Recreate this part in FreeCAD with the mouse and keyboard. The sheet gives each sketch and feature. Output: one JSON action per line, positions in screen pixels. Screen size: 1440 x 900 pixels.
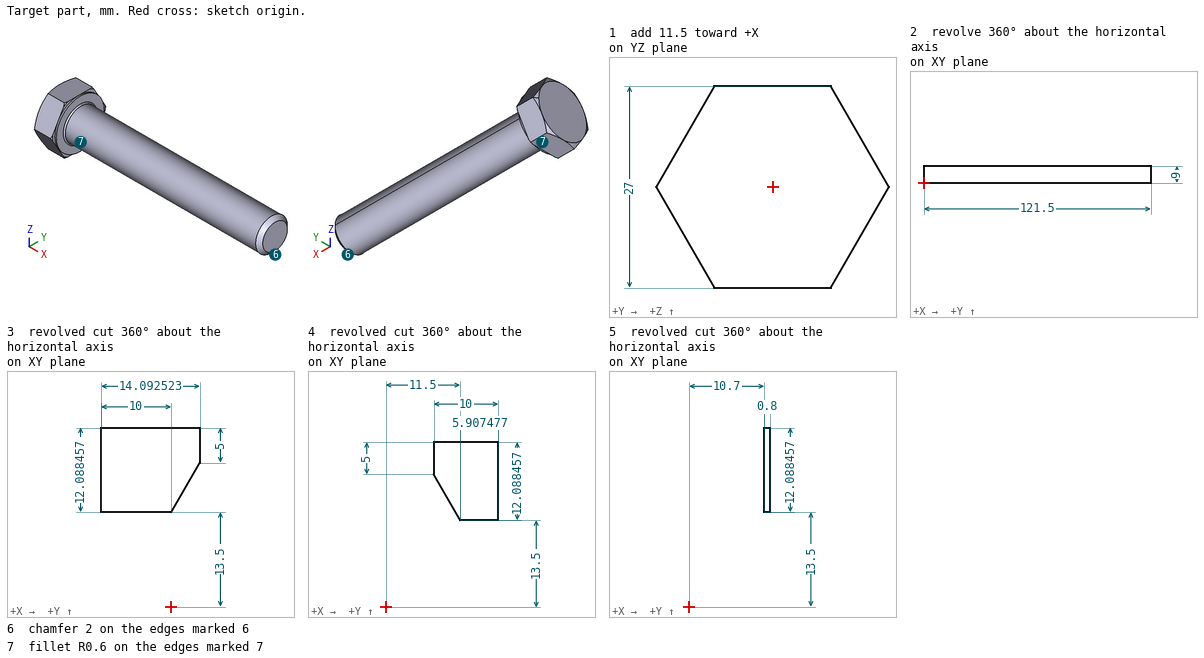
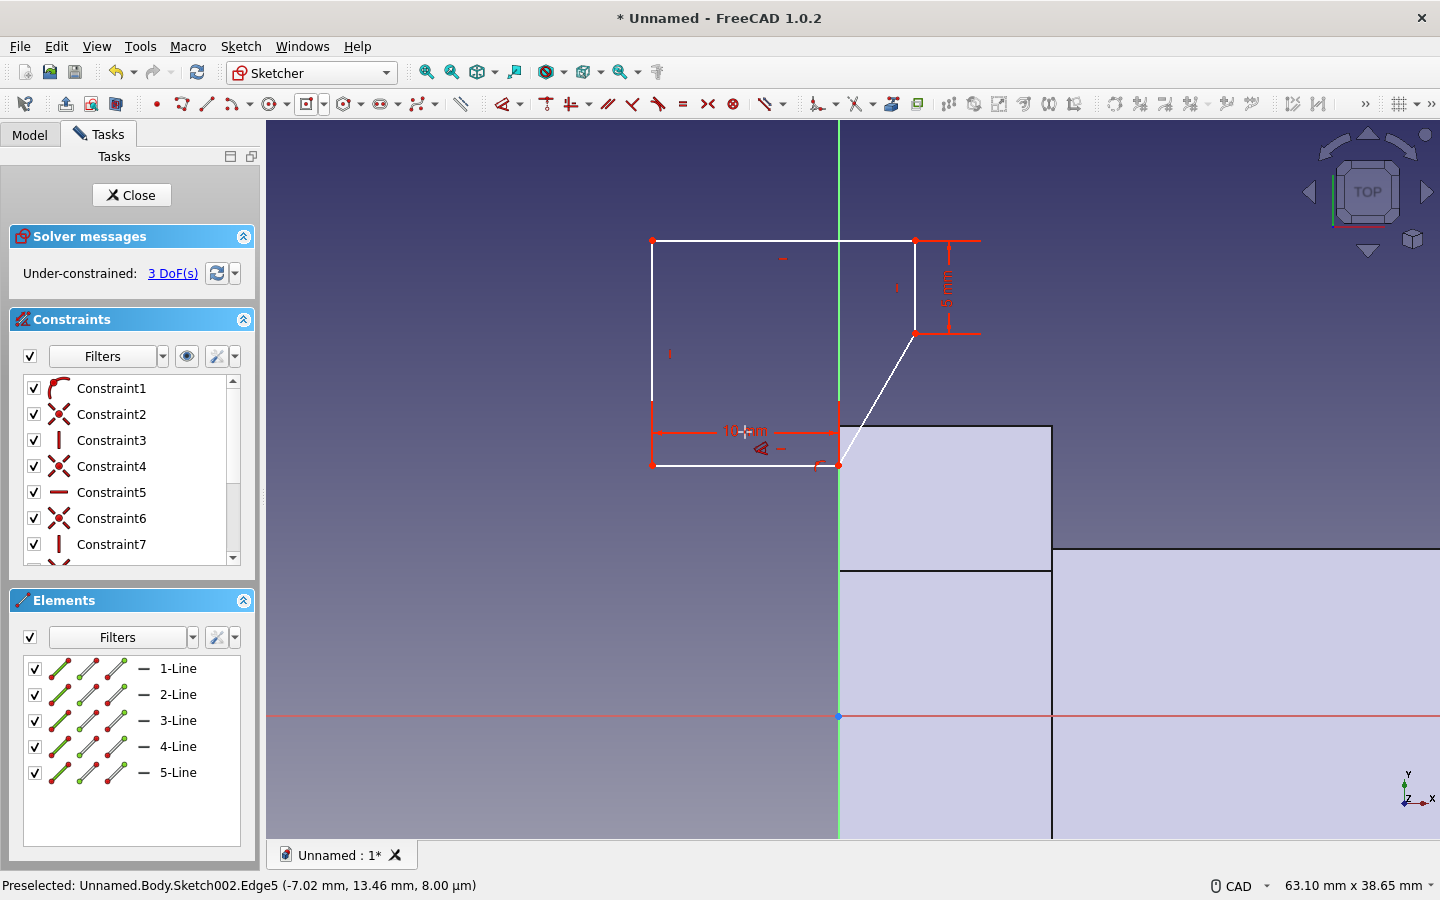
{"action": "left_click", "coordinate": [839, 466]}
{"action": "left_click", "coordinate": [873, 591]}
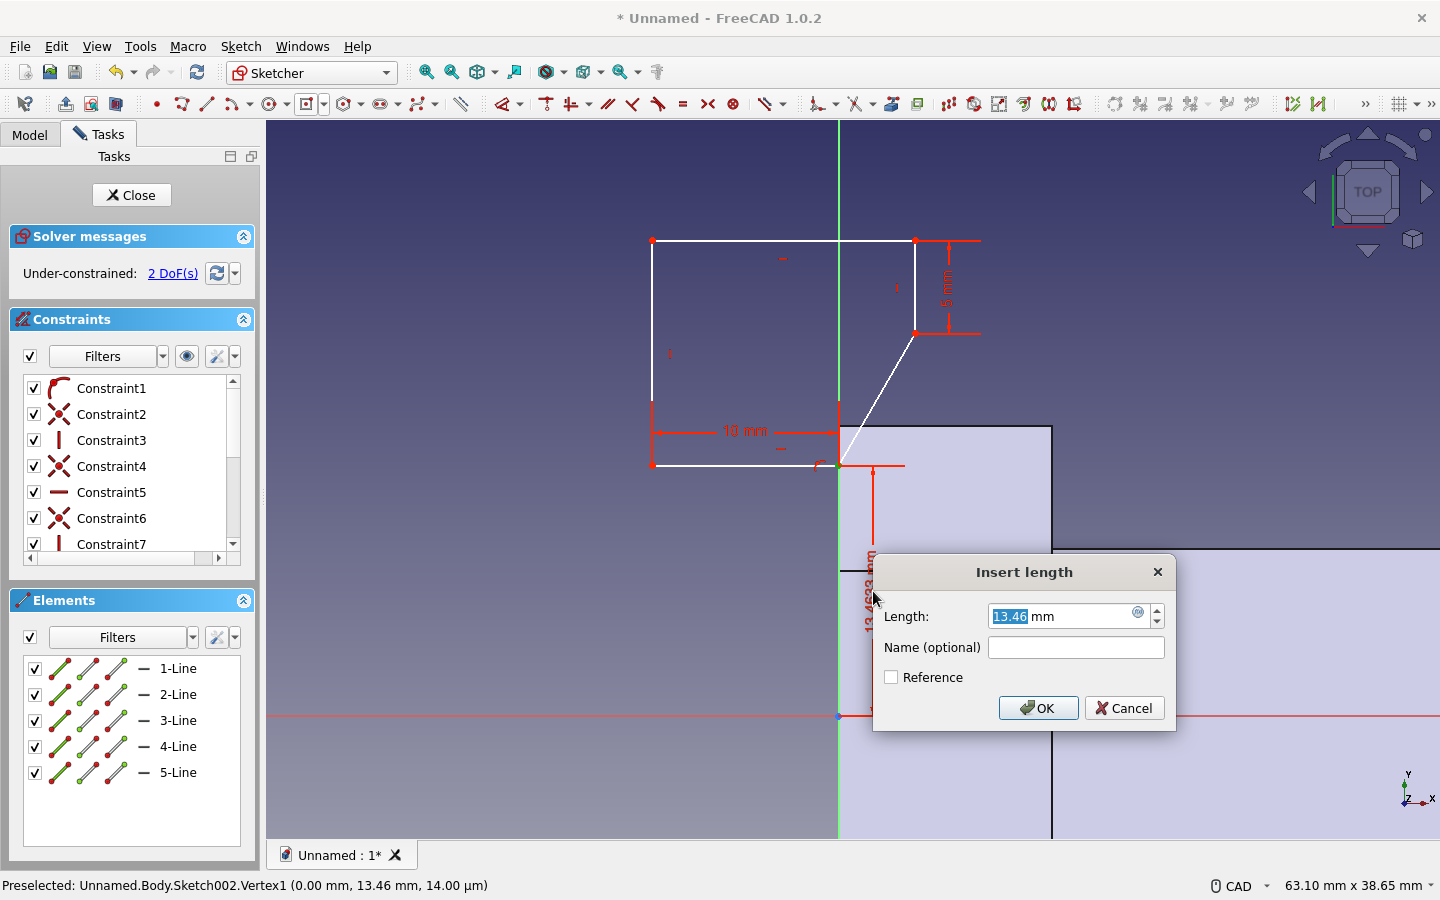
{"action": "type", "text": "13.5"}
{"action": "key", "text": "Return"}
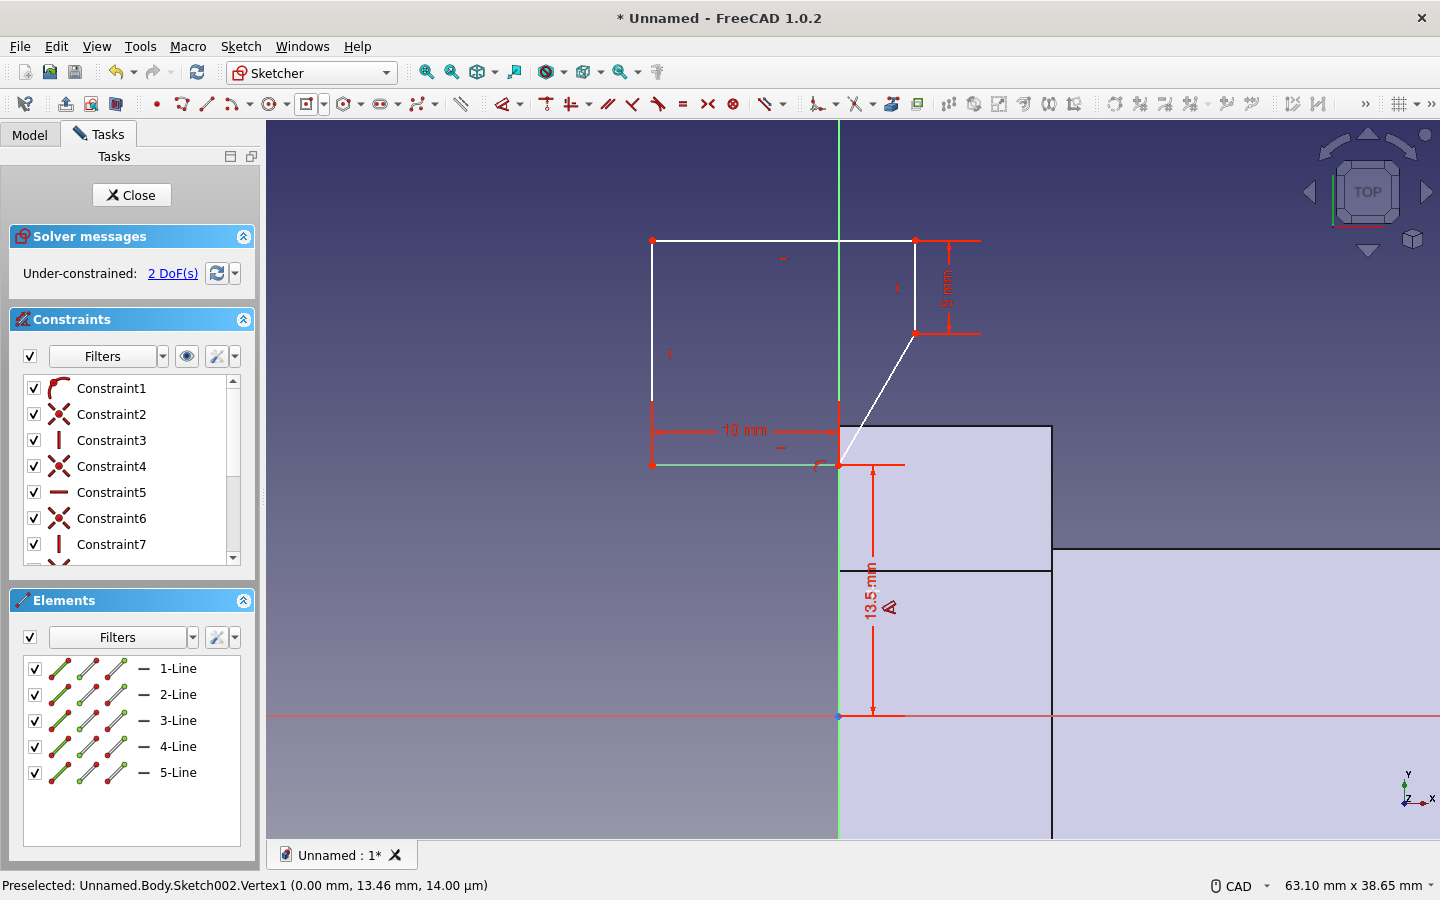
{"action": "left_click", "coordinate": [836, 241]}
{"action": "left_click", "coordinate": [784, 207]}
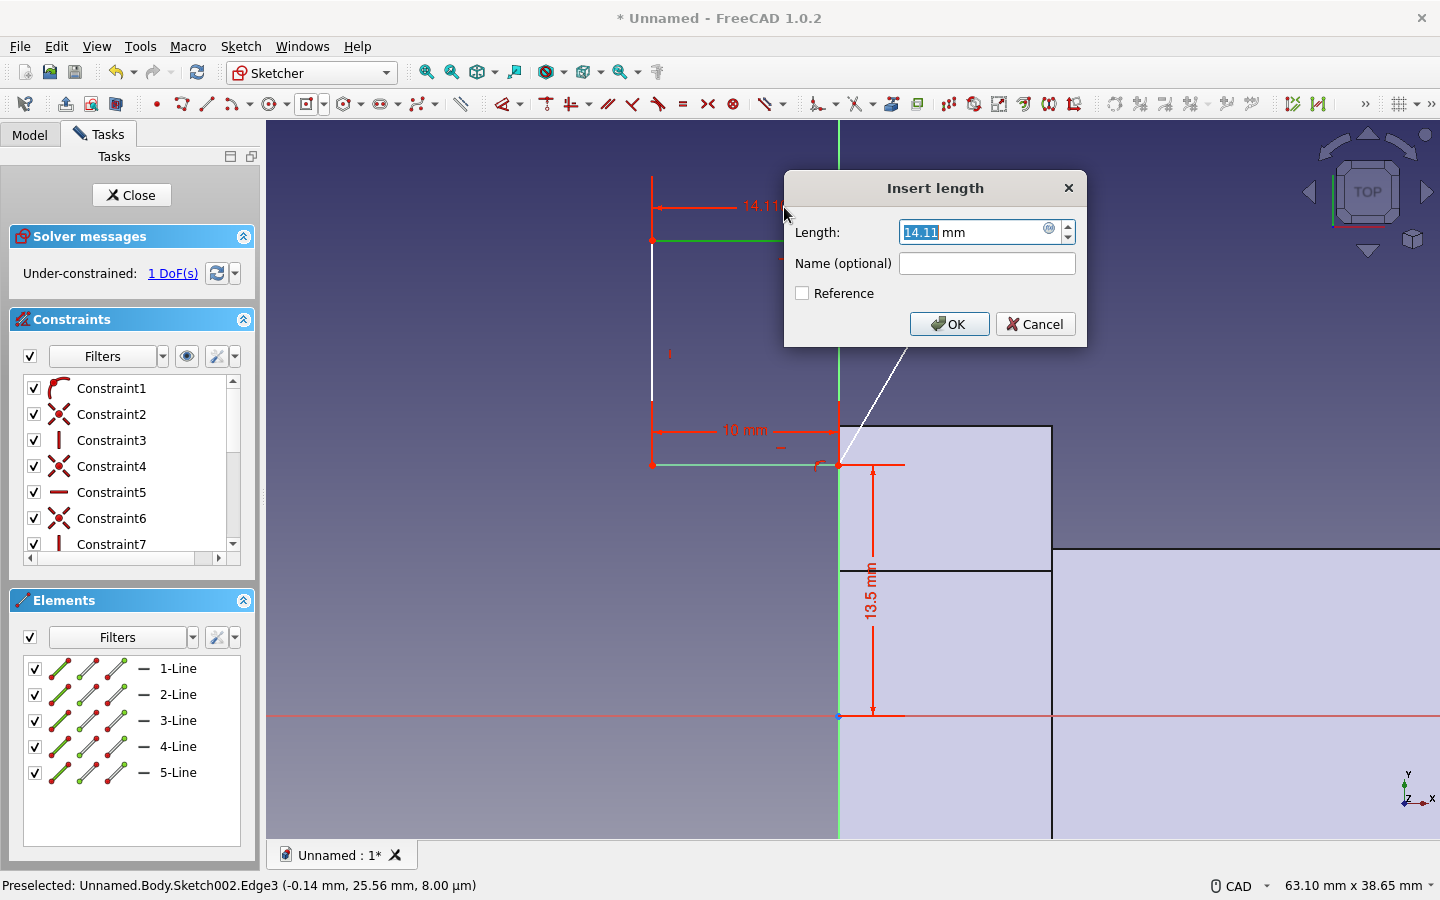
{"action": "type", "text": "14.092523"}
{"action": "key", "text": "Return"}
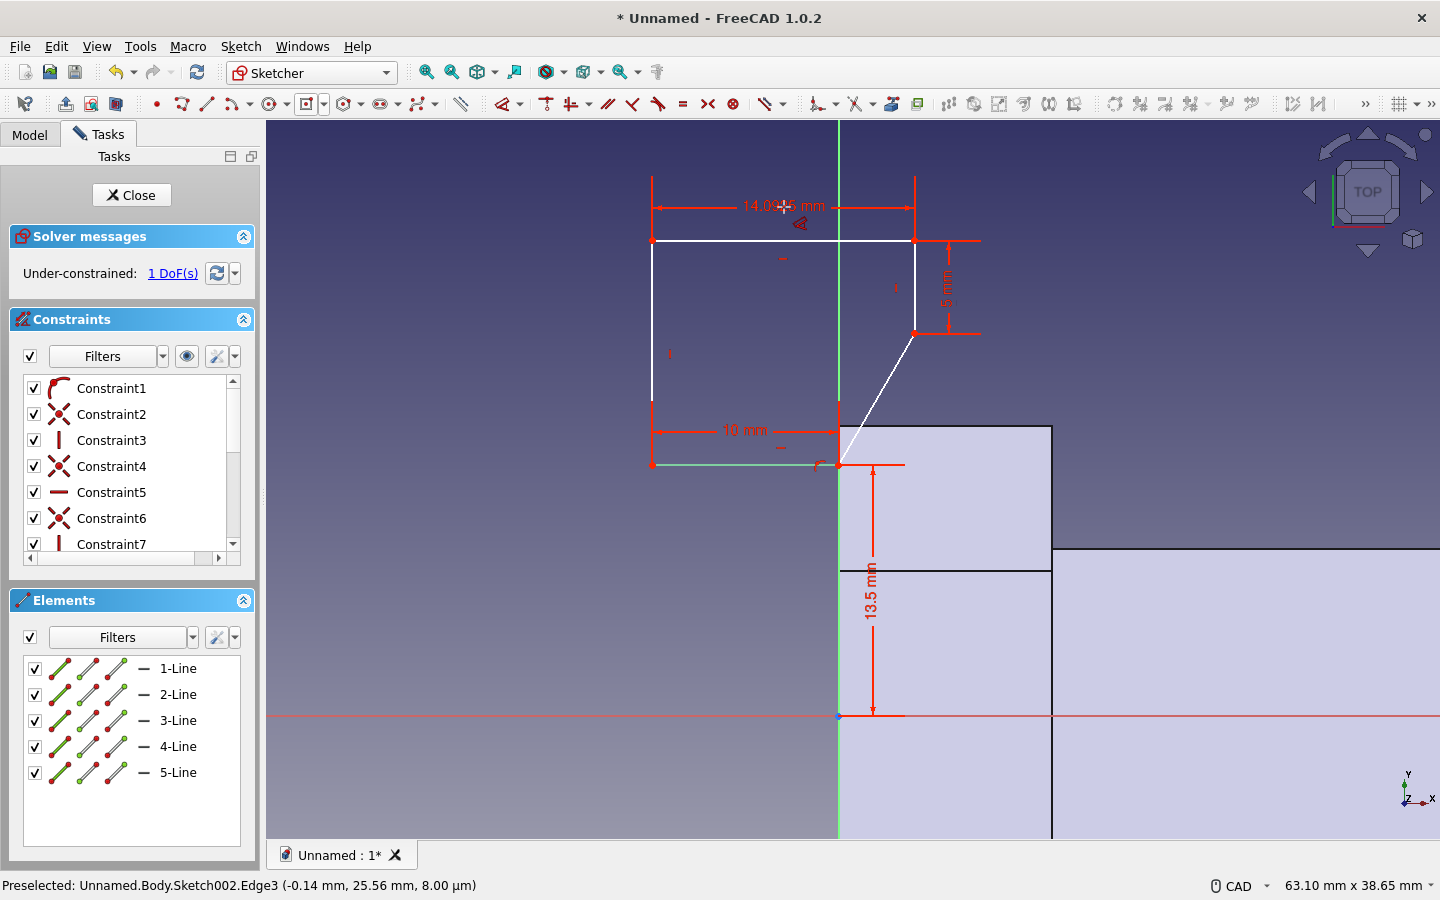
{"action": "left_click", "coordinate": [652, 308]}
{"action": "left_click", "coordinate": [618, 353]}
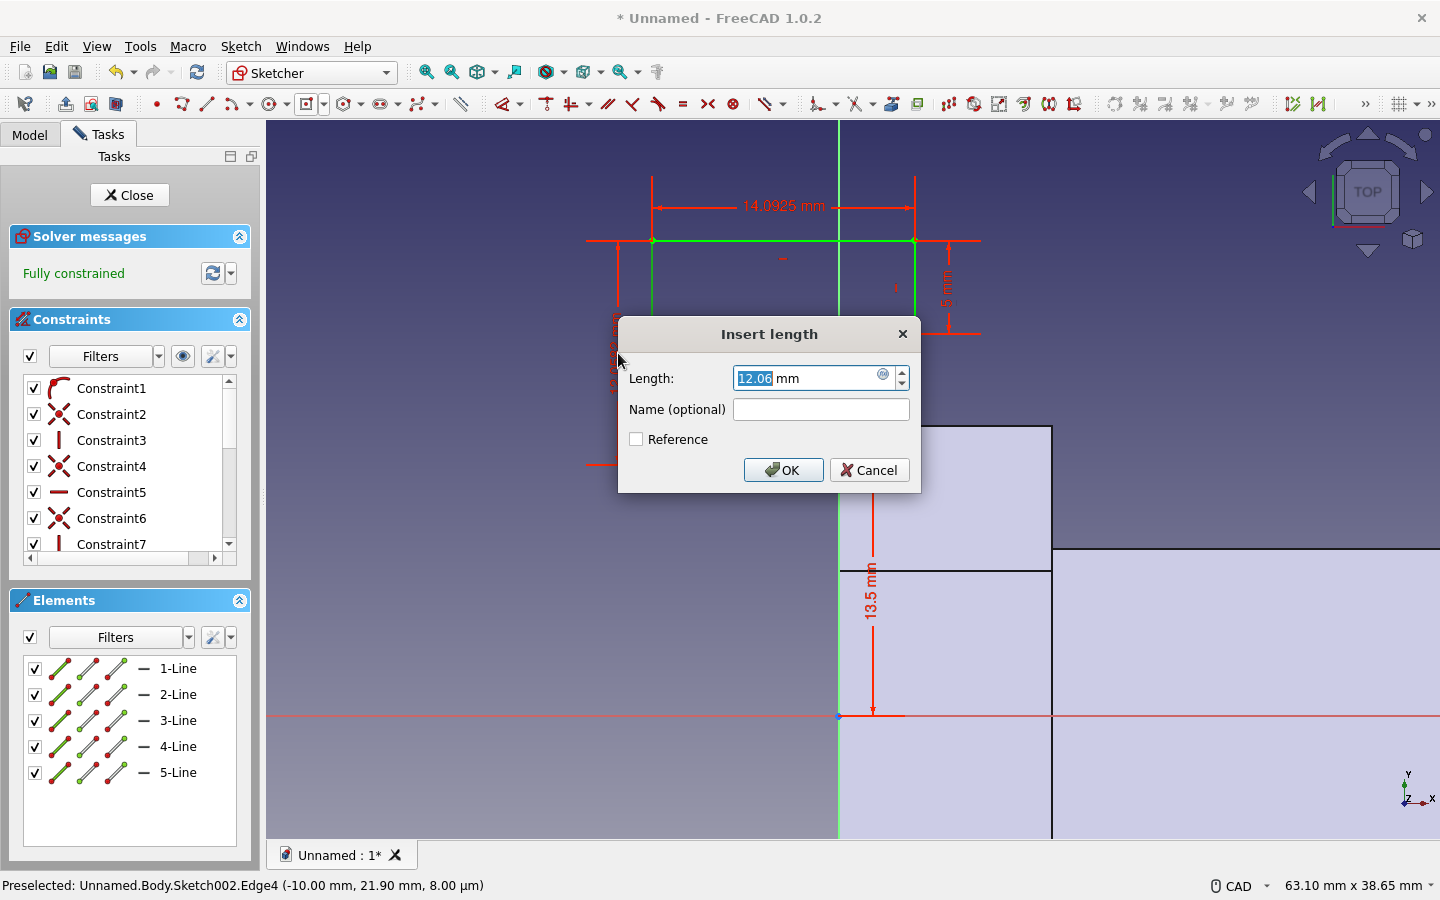
{"action": "type", "text": "12.088457"}
{"action": "key", "text": "Return"}
{"action": "key", "text": "Escape"}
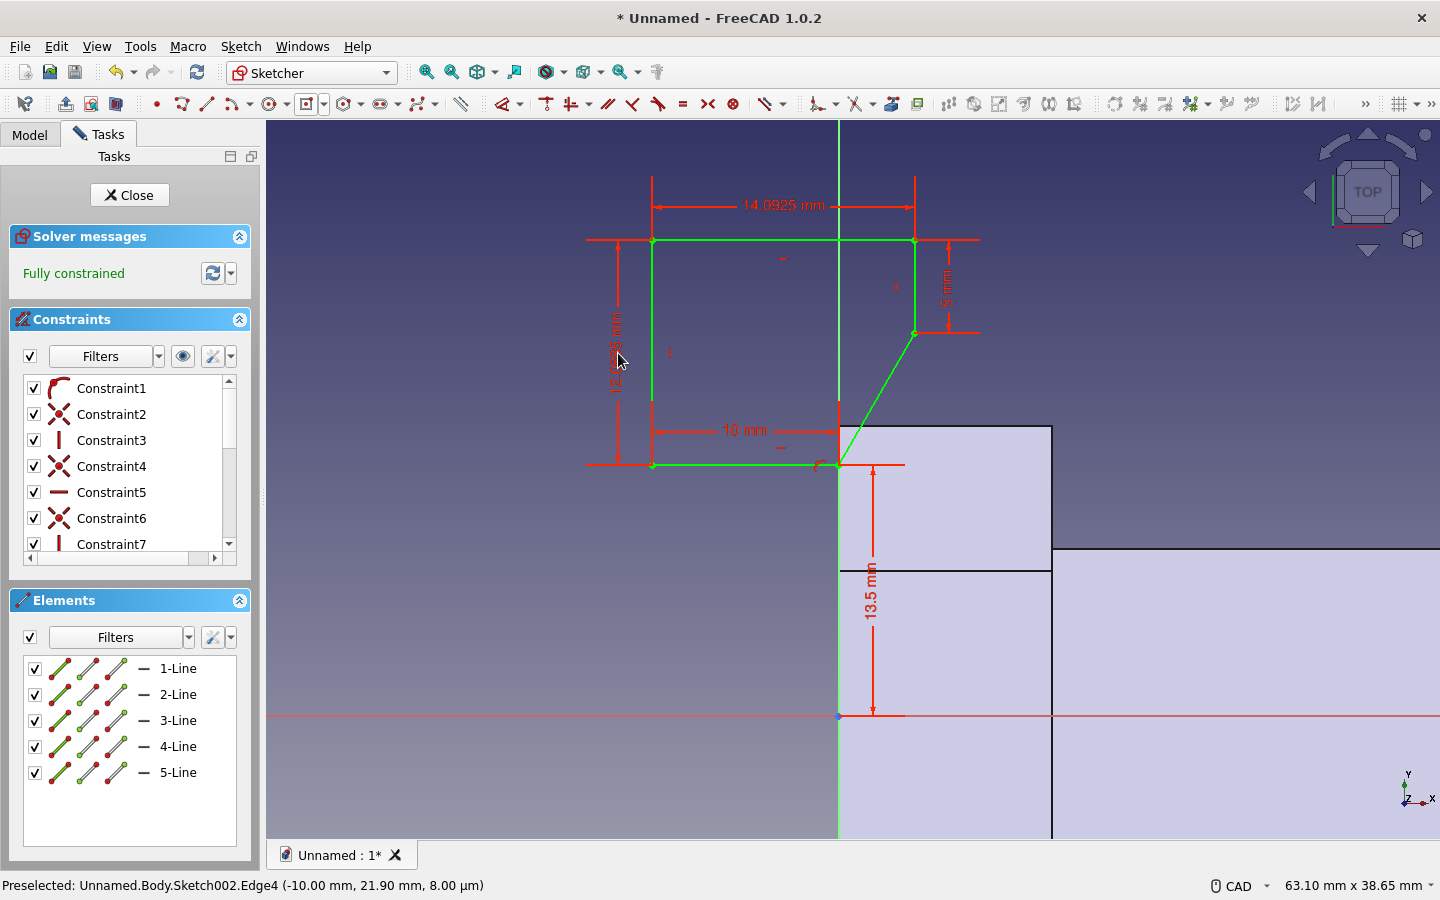
{"action": "left_click", "coordinate": [130, 195]}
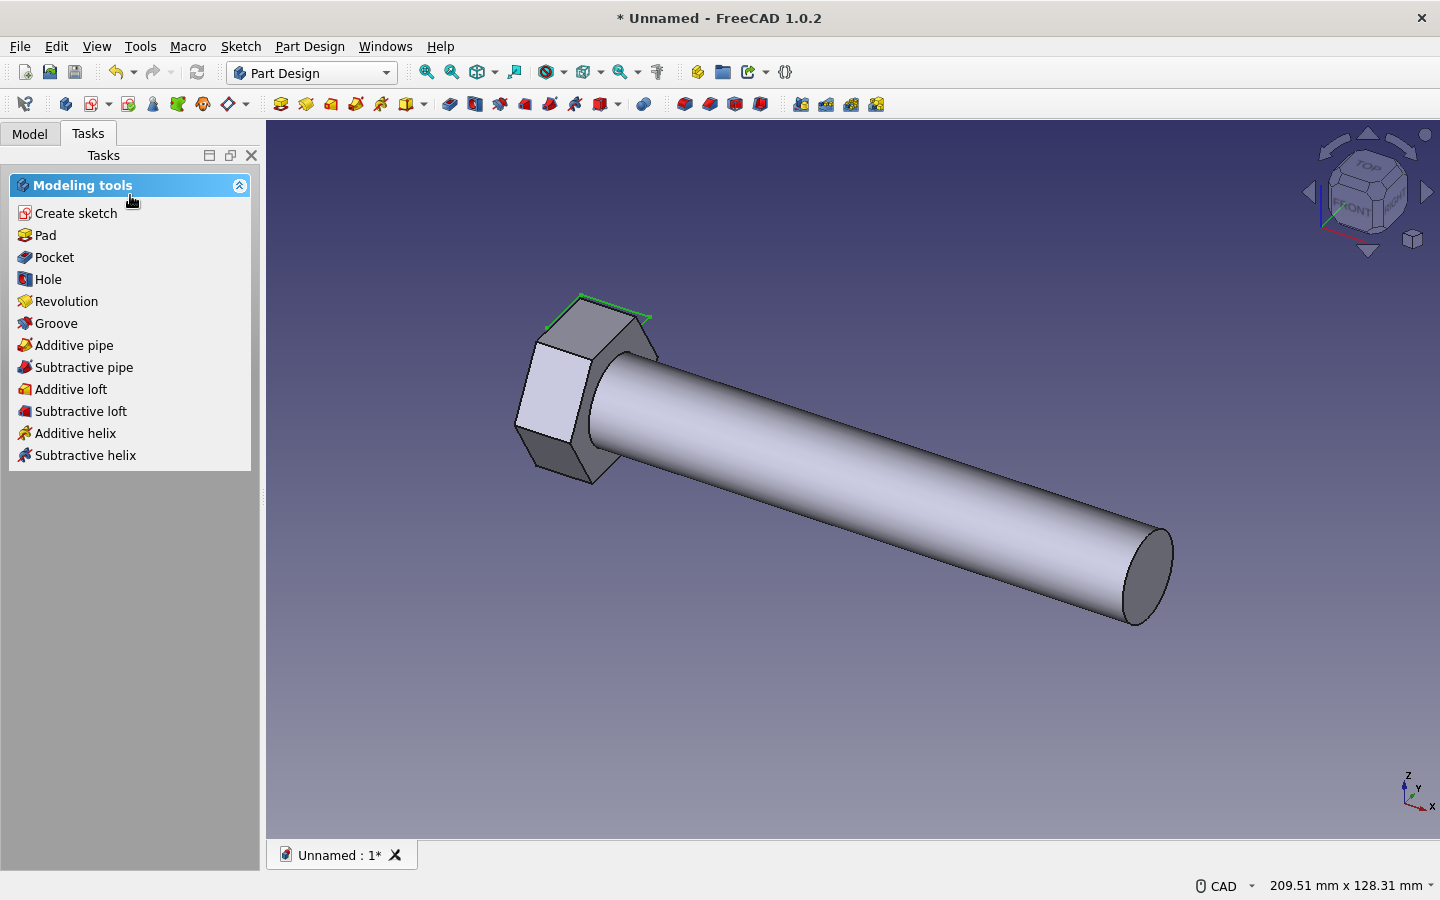
{"action": "left_click", "coordinate": [500, 104]}